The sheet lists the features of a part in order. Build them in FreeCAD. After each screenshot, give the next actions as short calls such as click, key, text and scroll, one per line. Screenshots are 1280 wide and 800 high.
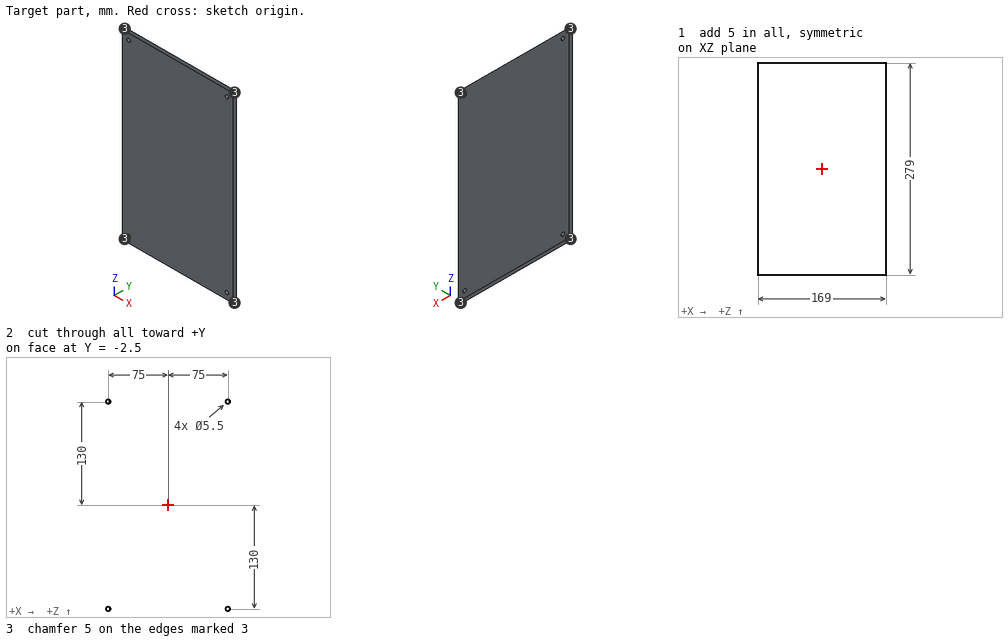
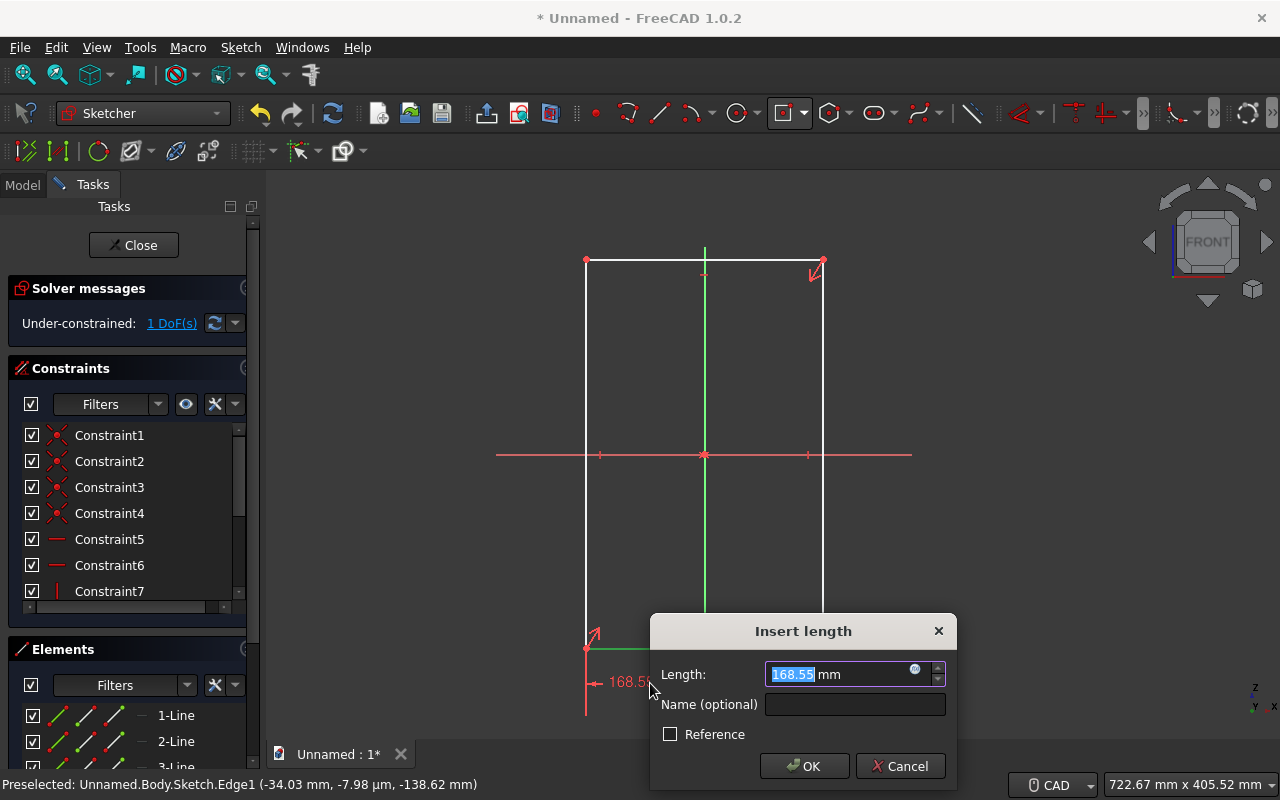
text(169)
key(Return)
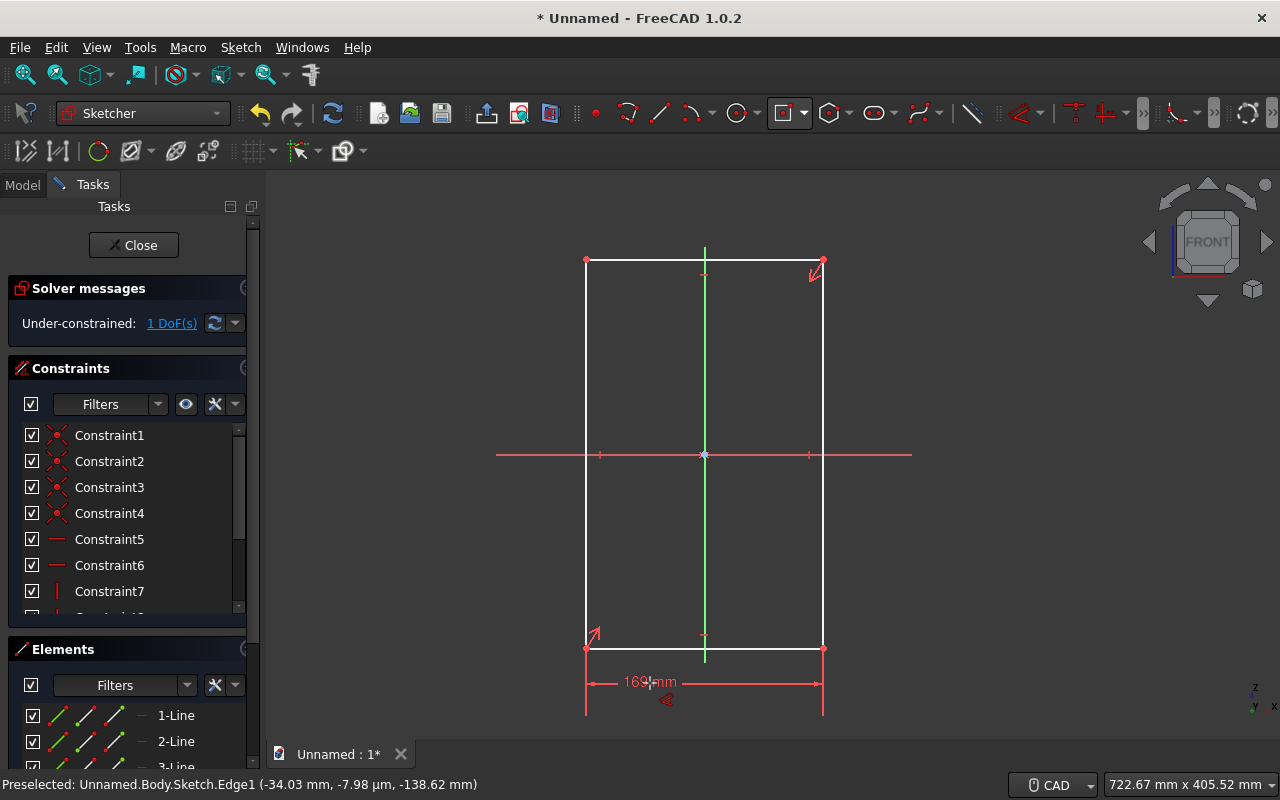
click(823, 532)
click(857, 365)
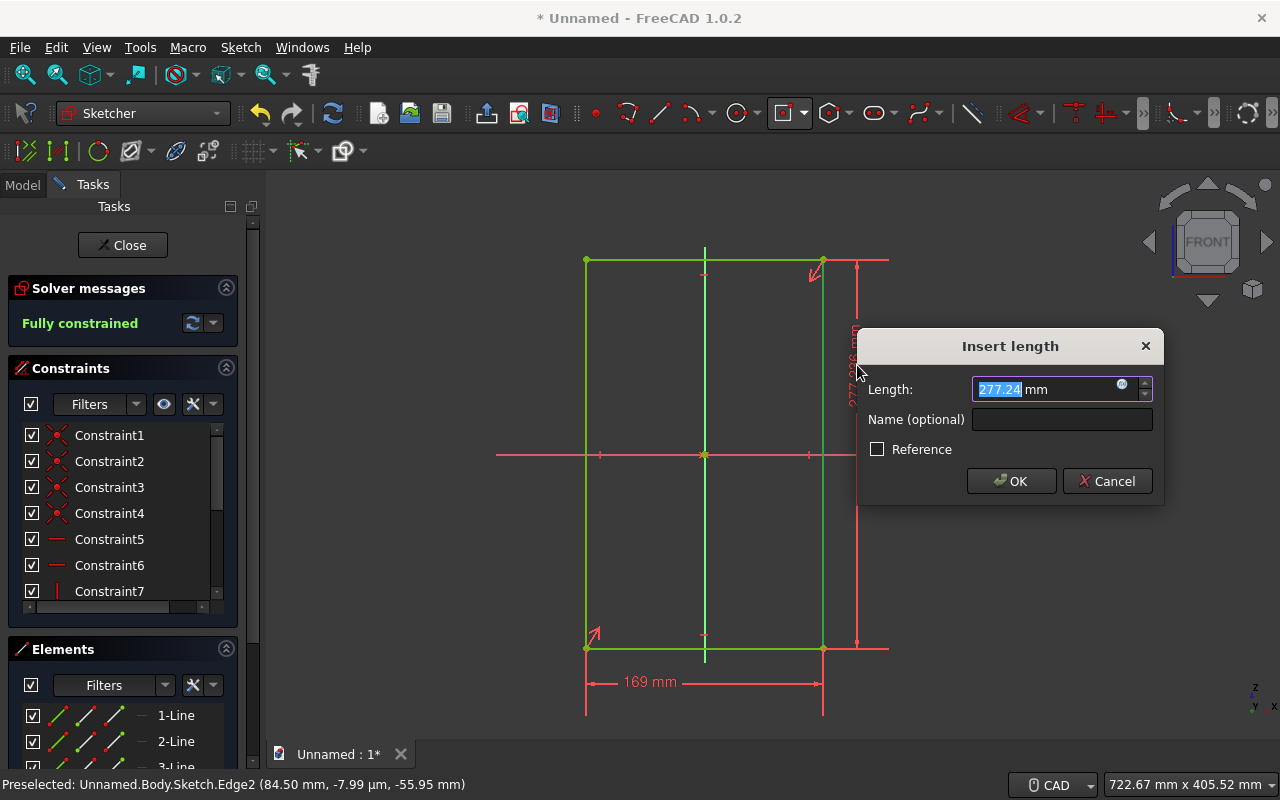
text(279)
key(Return)
key(Escape)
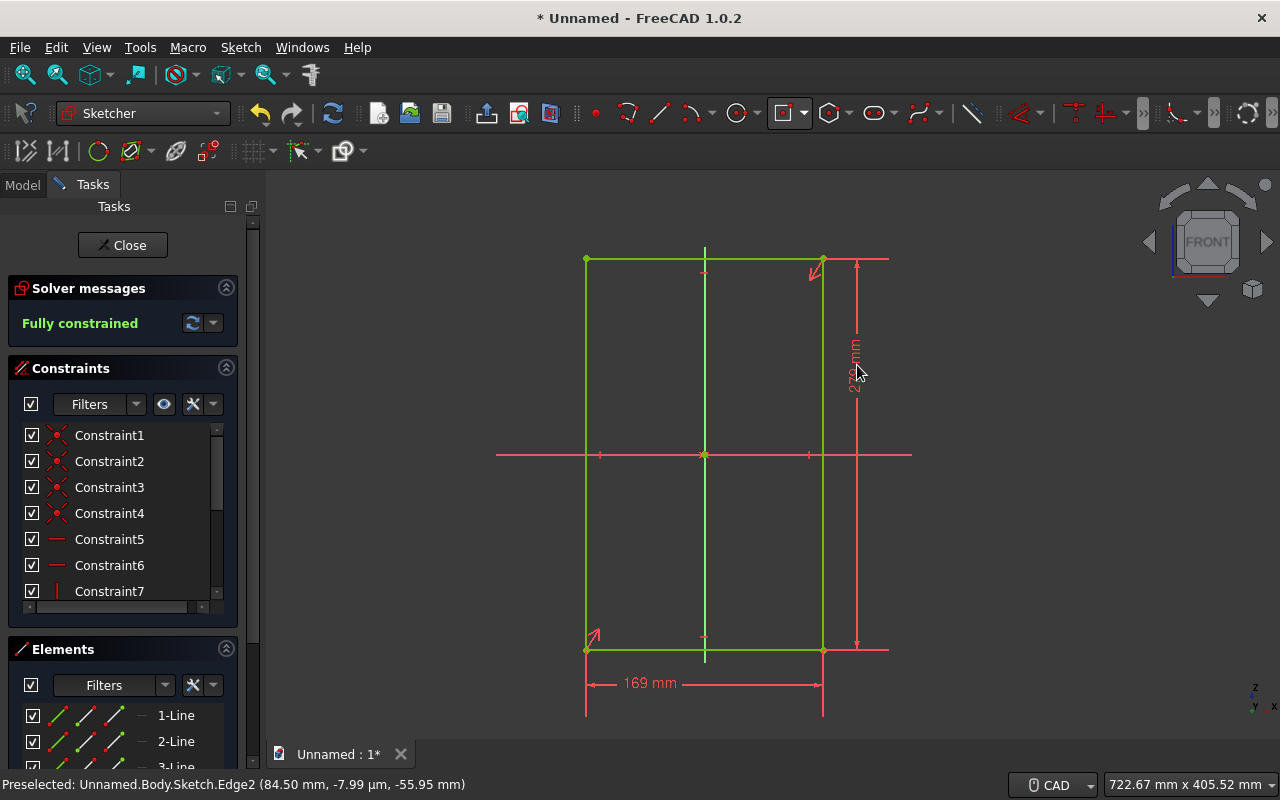
click(123, 245)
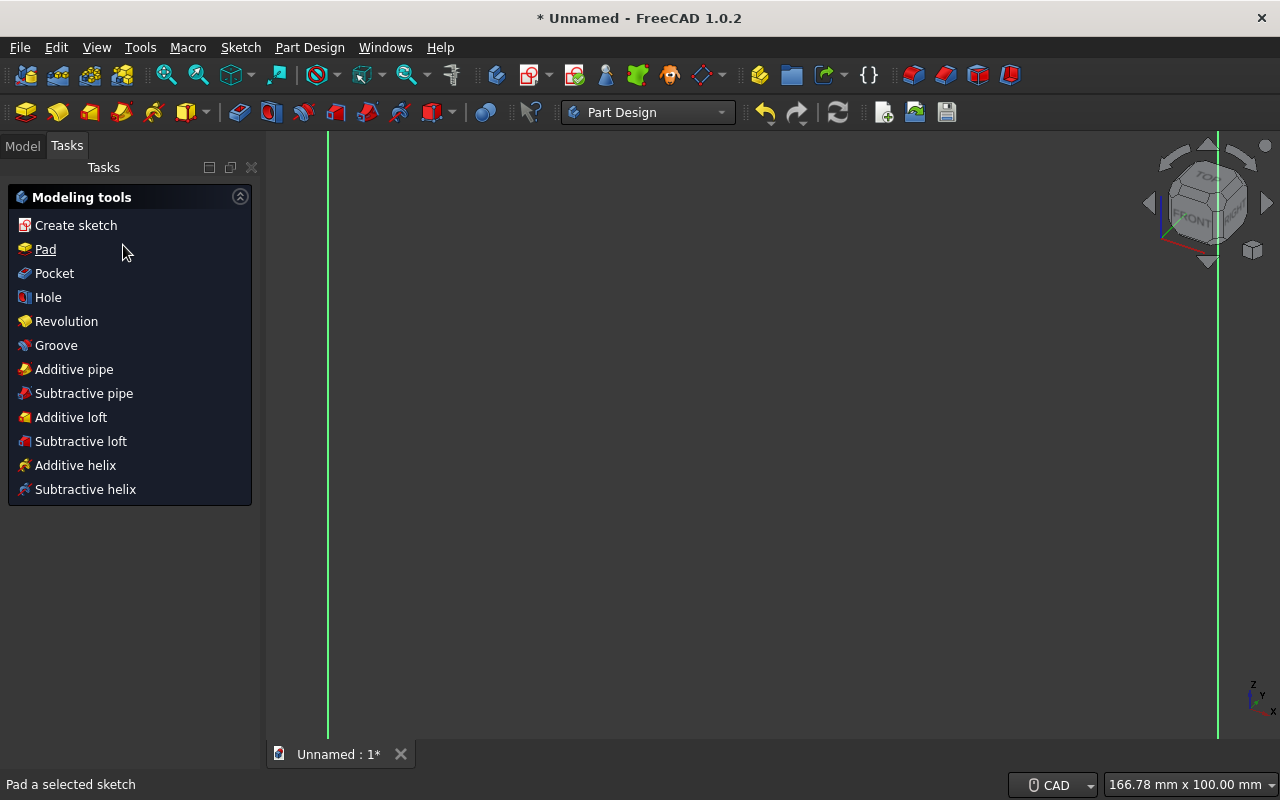
click(26, 112)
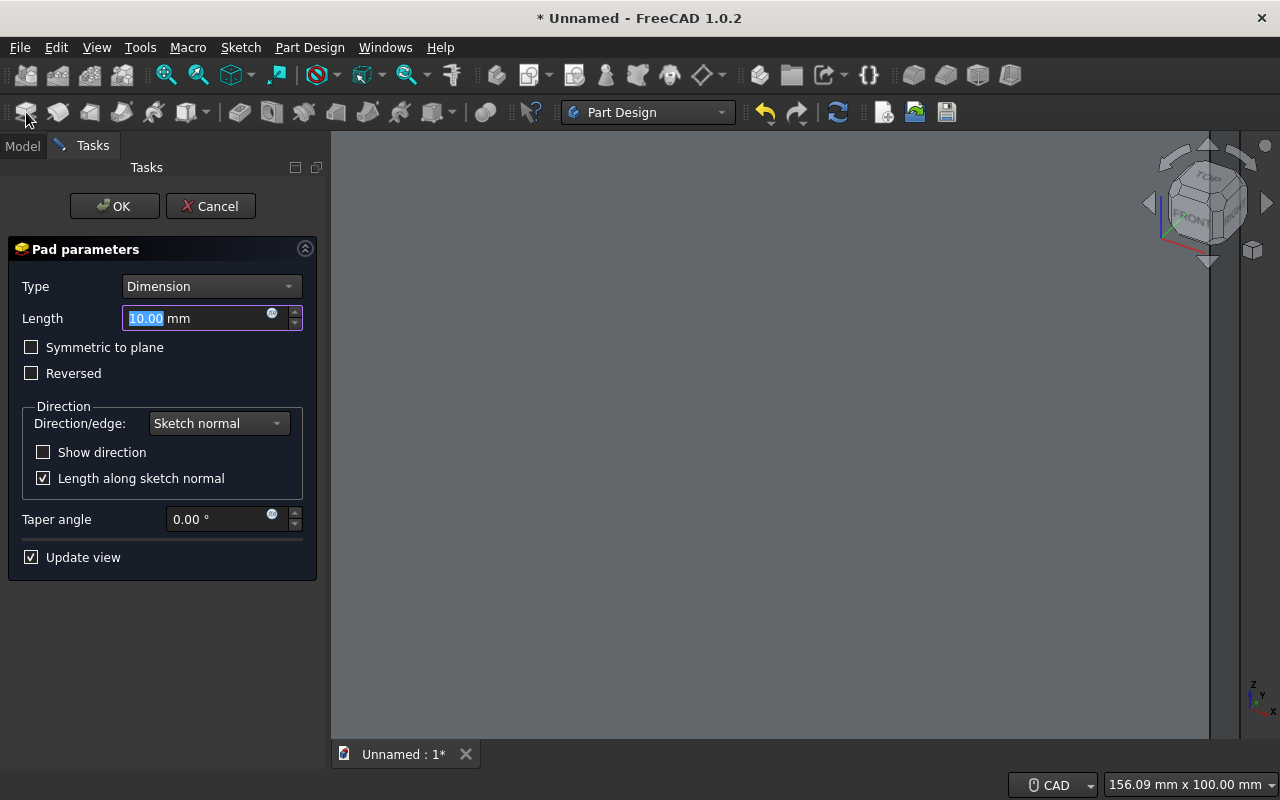
text(5)
key(Tab)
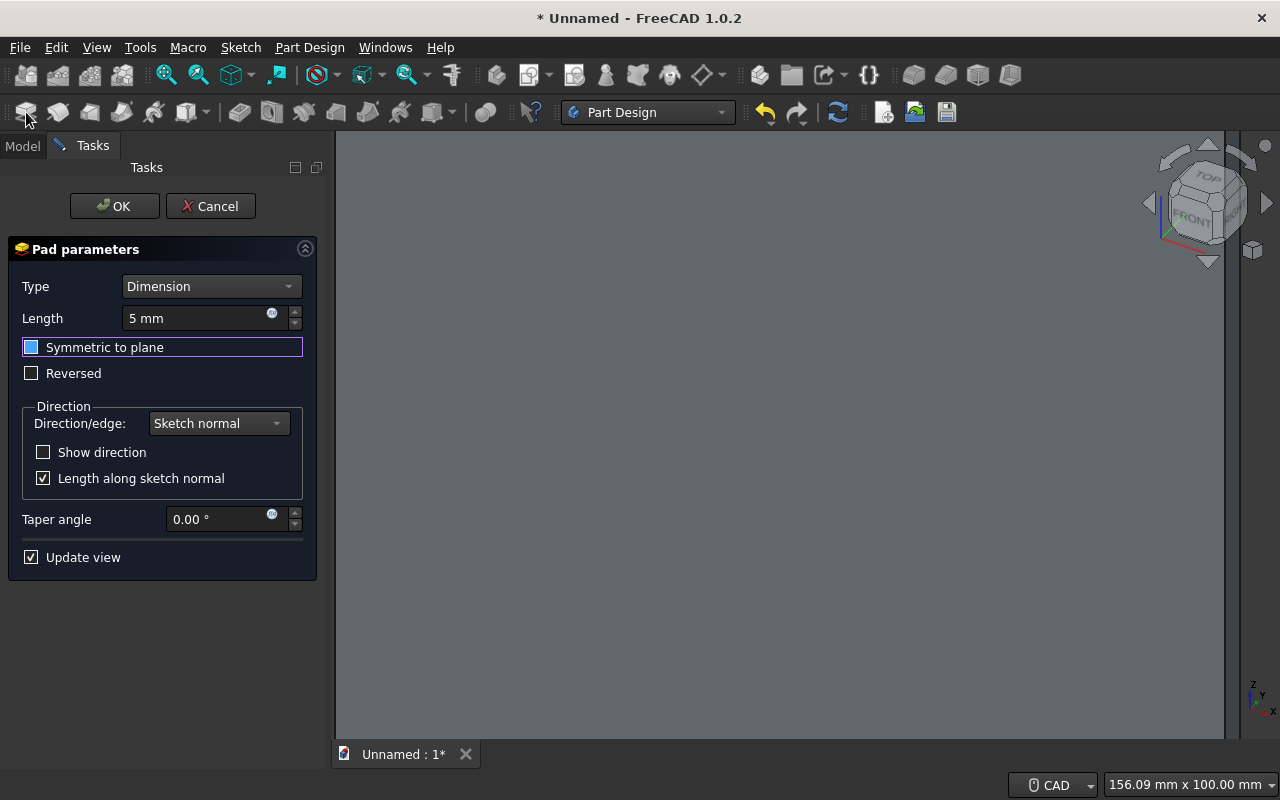
click(30, 347)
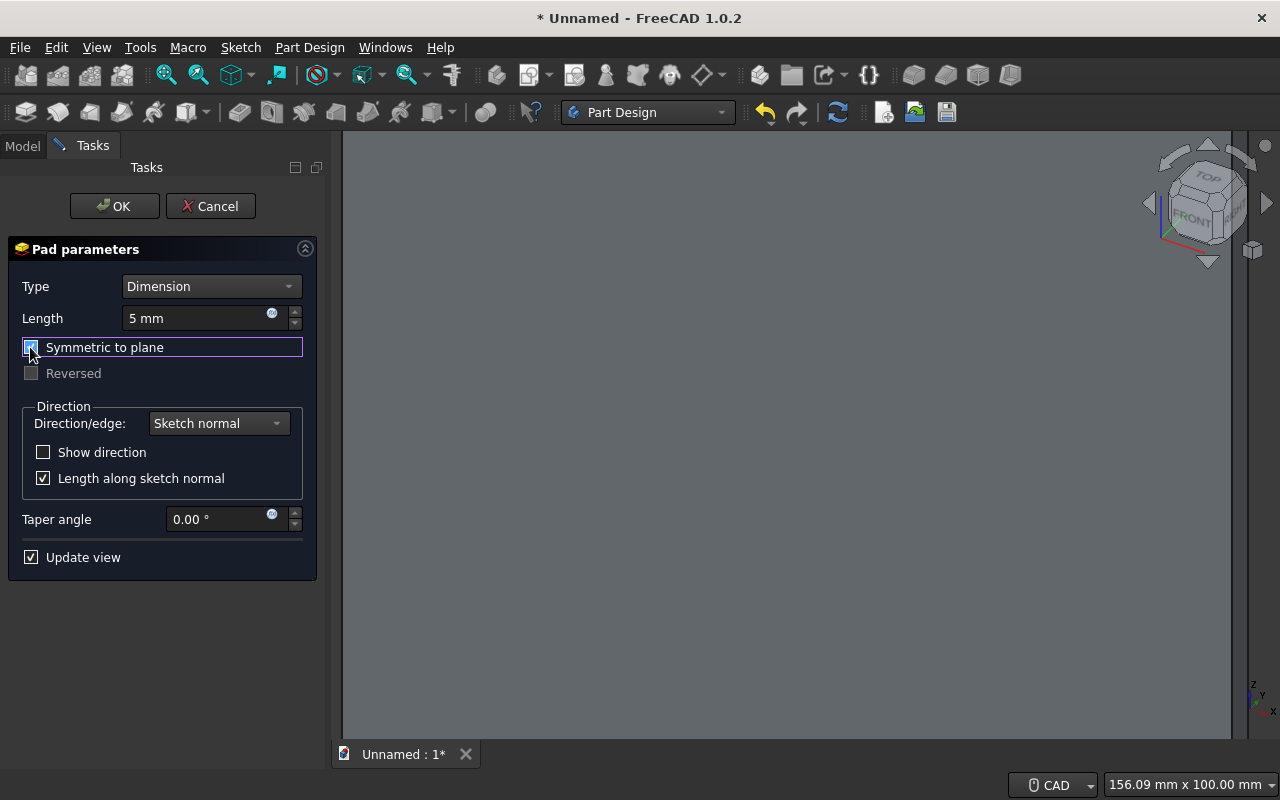
click(115, 206)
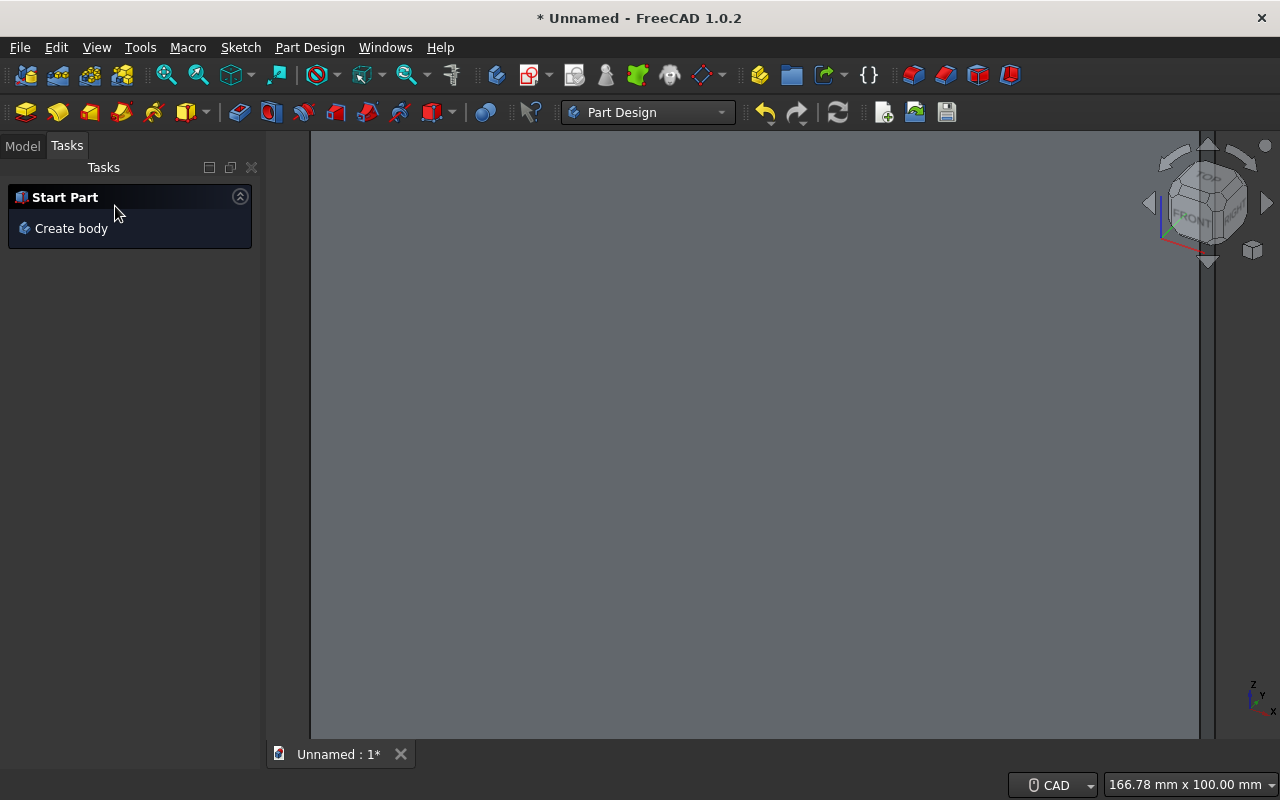
click(168, 76)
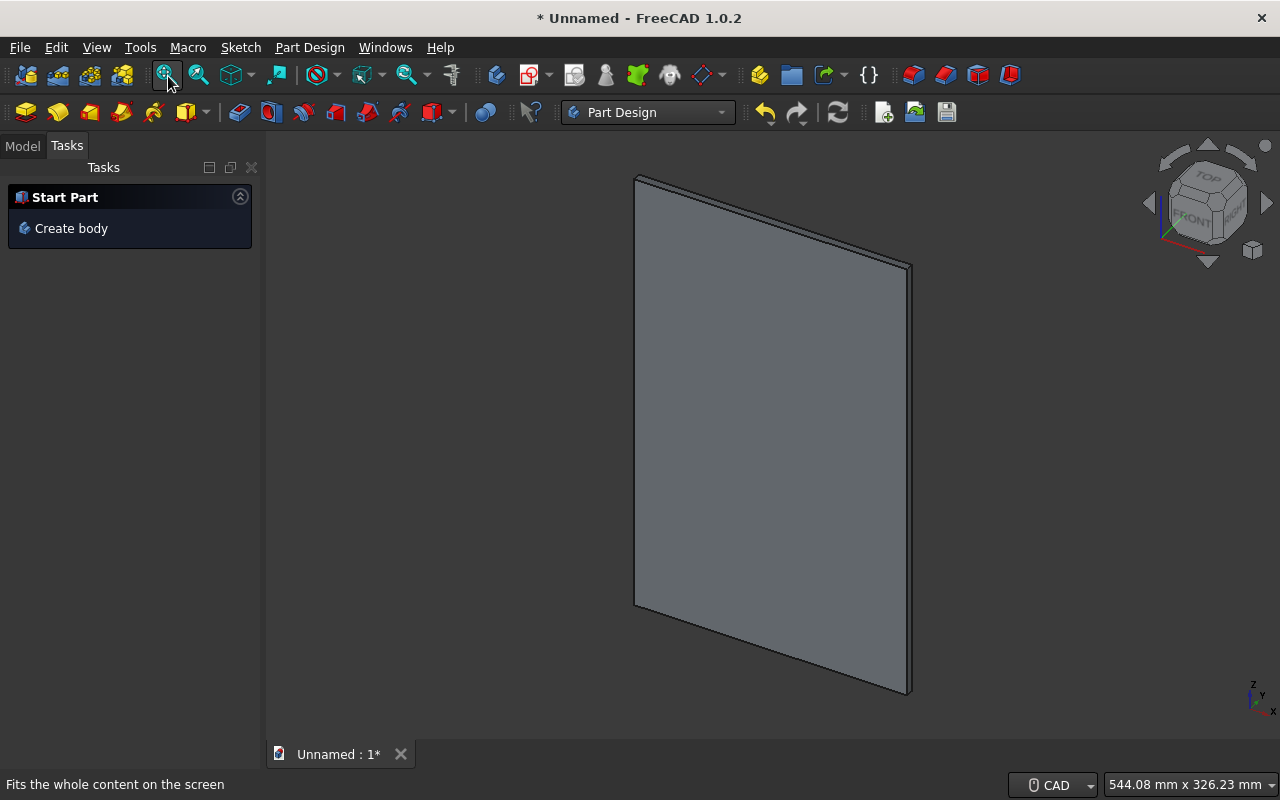
click(771, 375)